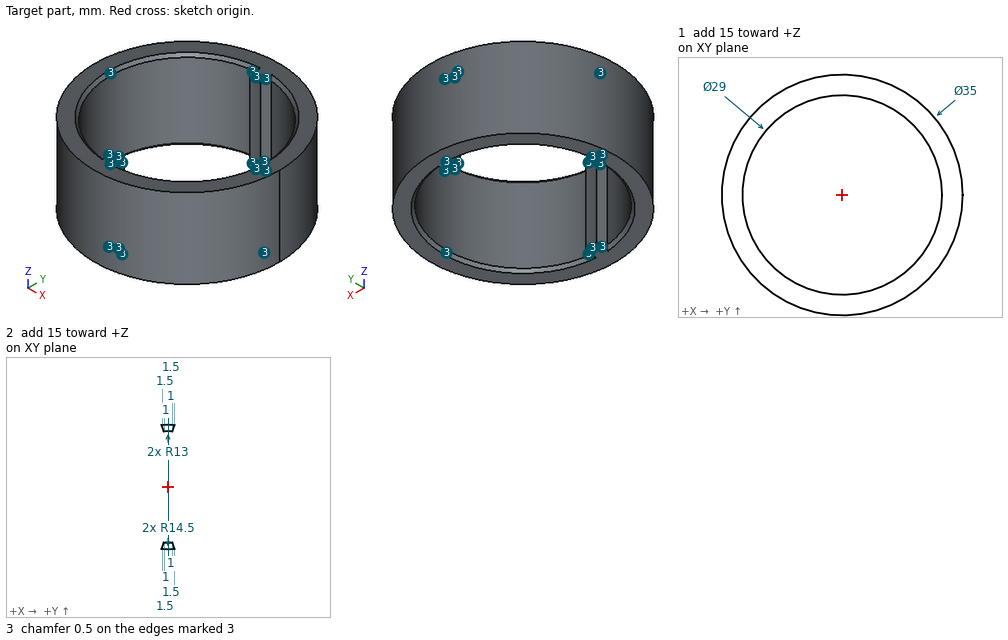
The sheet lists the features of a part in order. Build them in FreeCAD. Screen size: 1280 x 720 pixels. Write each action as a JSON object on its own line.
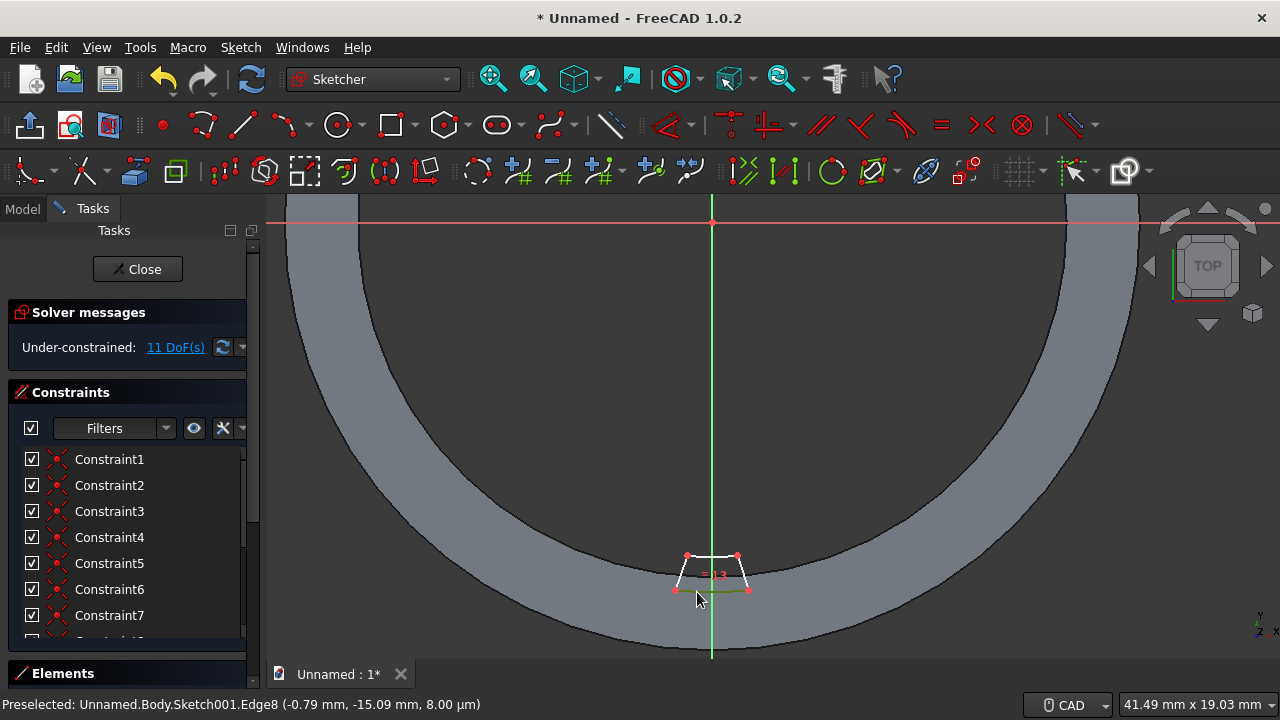
{"action": "left_click", "coordinate": [942, 126]}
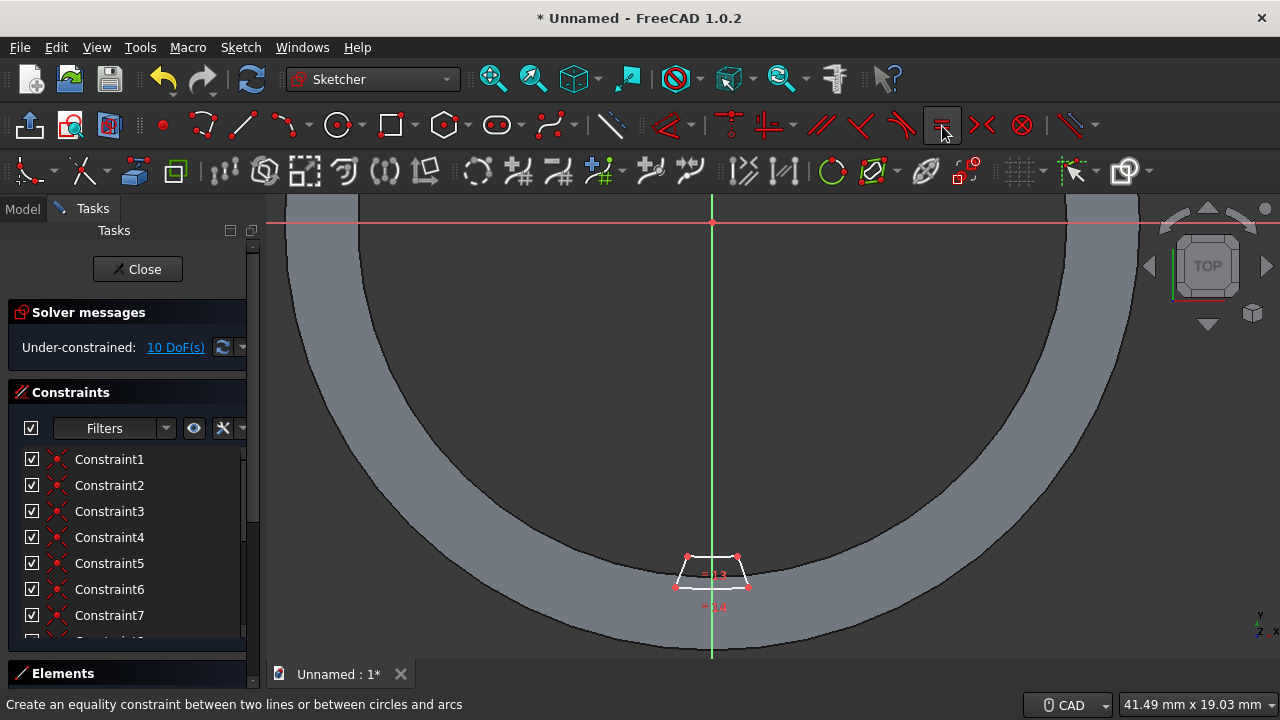
{"action": "key", "text": "d"}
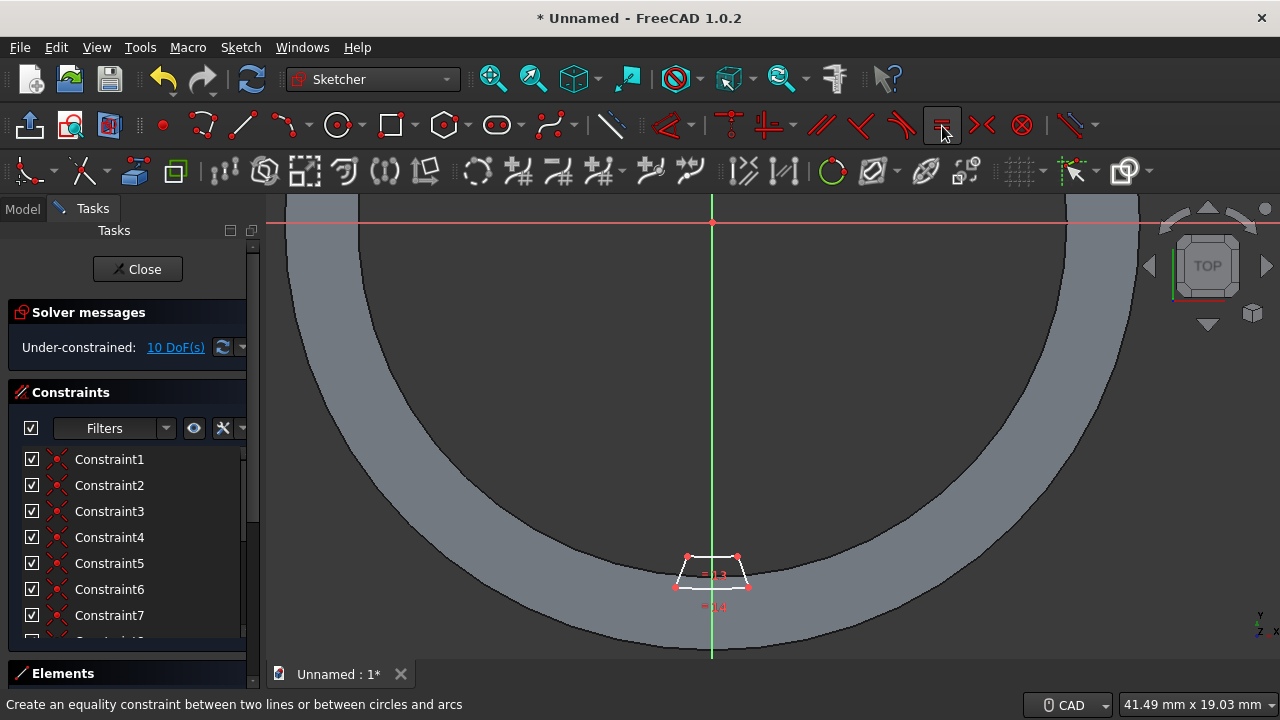
{"action": "scroll", "coordinate": [698, 593], "scroll_direction": "down", "scroll_amount": 4}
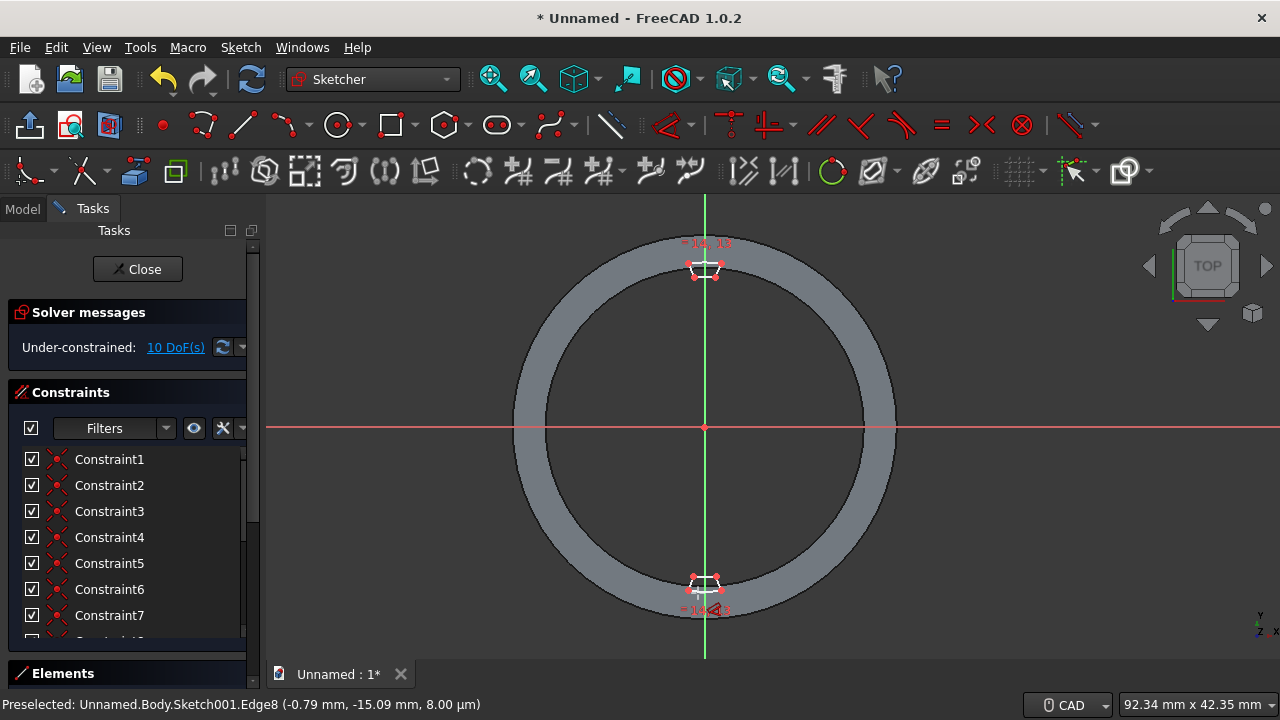
{"action": "scroll", "coordinate": [709, 277], "scroll_direction": "up", "scroll_amount": 6}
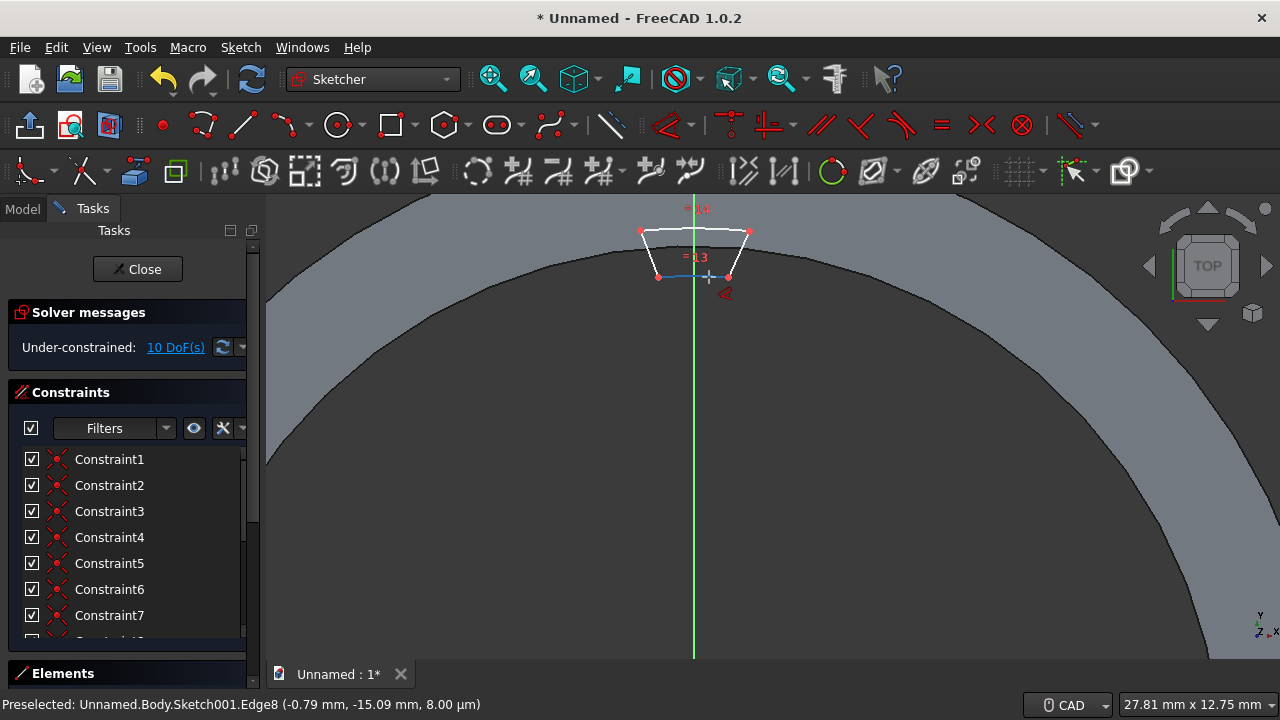
{"action": "left_click", "coordinate": [708, 276]}
{"action": "left_click", "coordinate": [709, 244]}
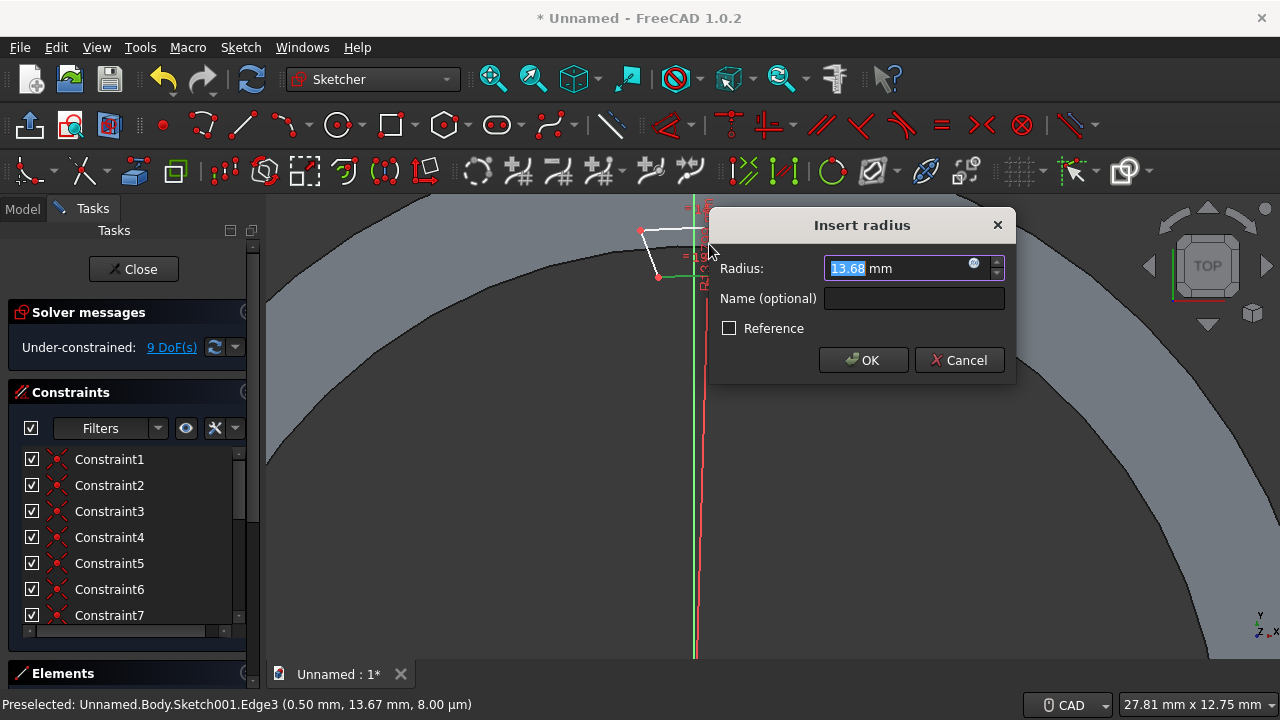
{"action": "type", "text": "13"}
{"action": "key", "text": "Return"}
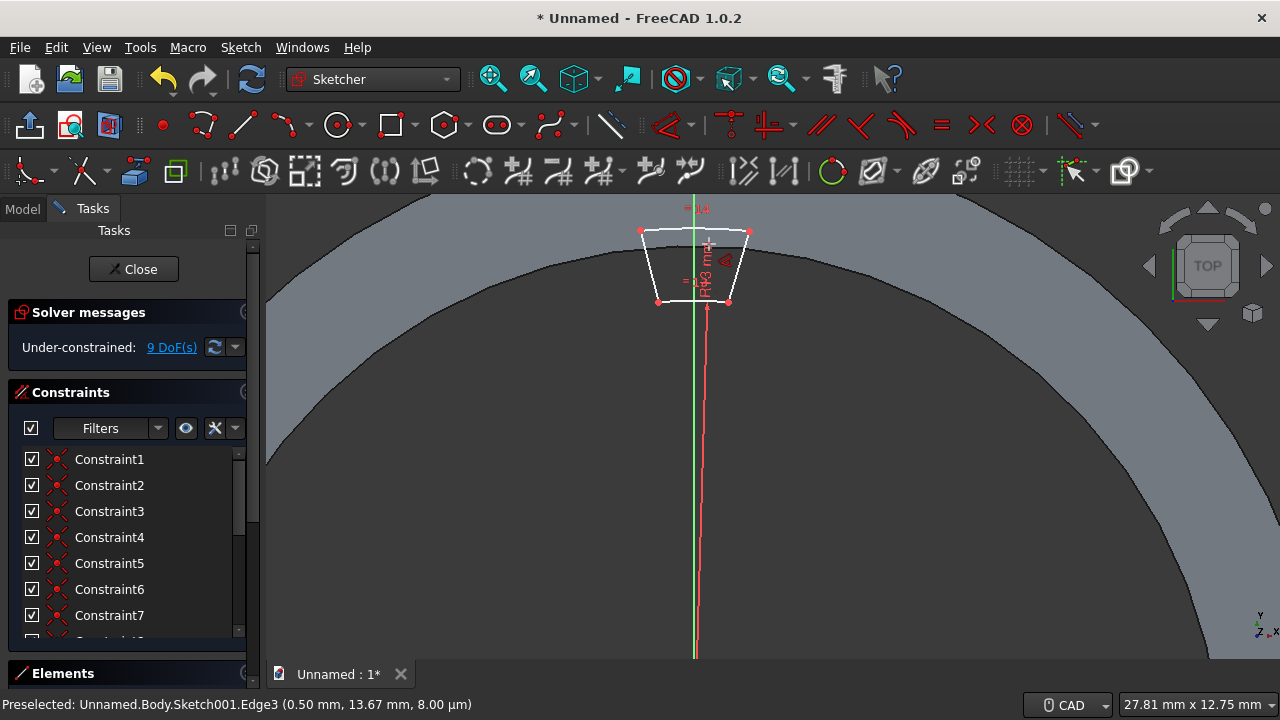
{"action": "left_click", "coordinate": [717, 229]}
{"action": "left_click", "coordinate": [992, 280]}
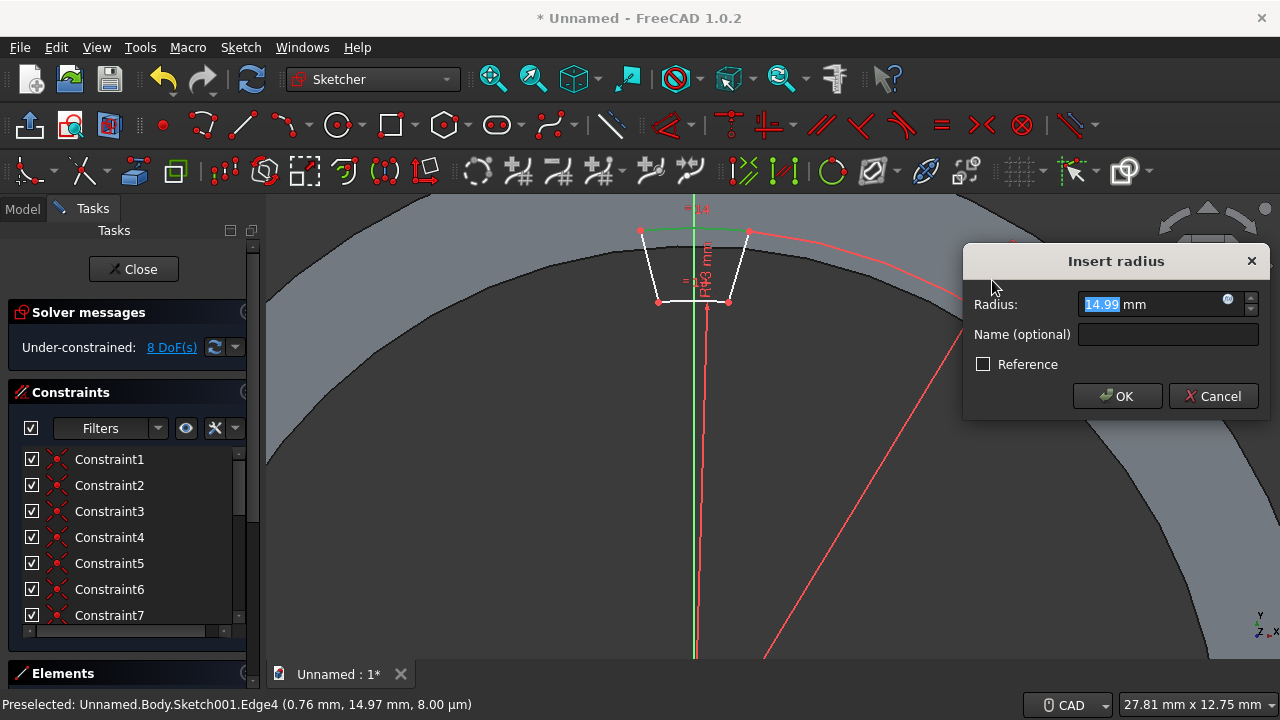
{"action": "type", "text": "14.5"}
{"action": "key", "text": "Return"}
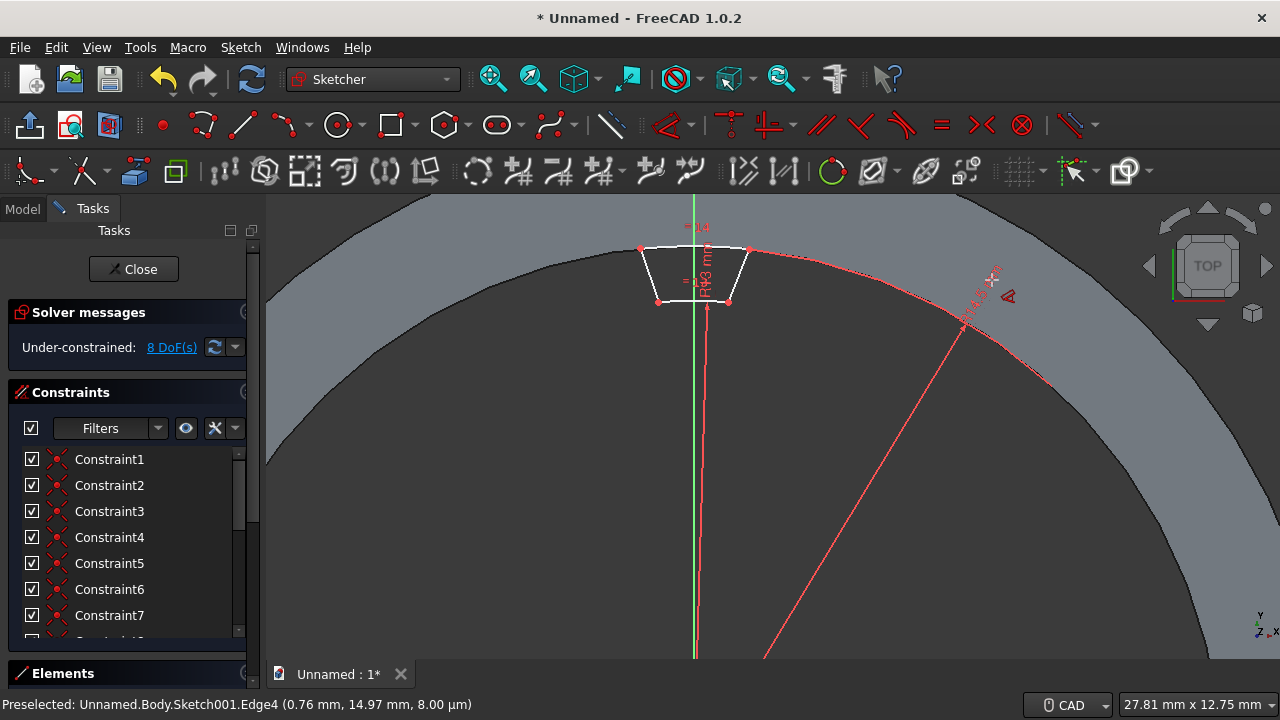
{"action": "left_click", "coordinate": [659, 302]}
{"action": "left_click", "coordinate": [676, 268]}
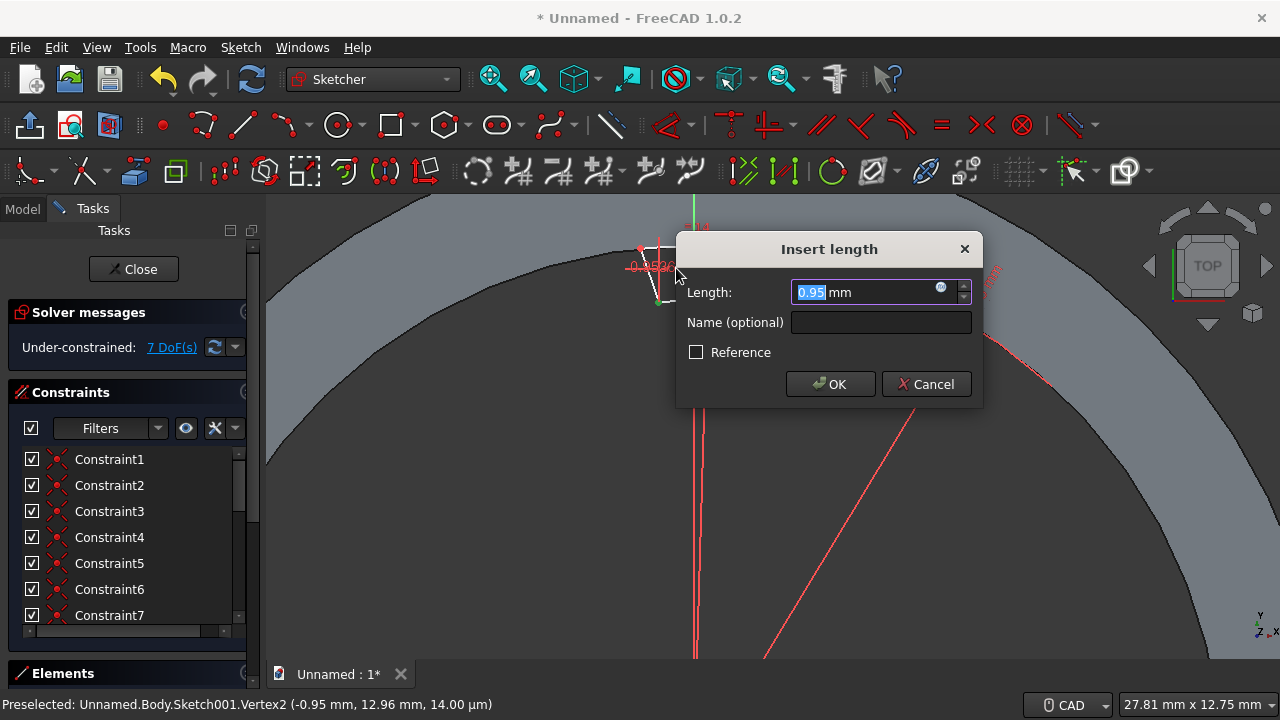
{"action": "type", "text": "1"}
{"action": "key", "text": "Return"}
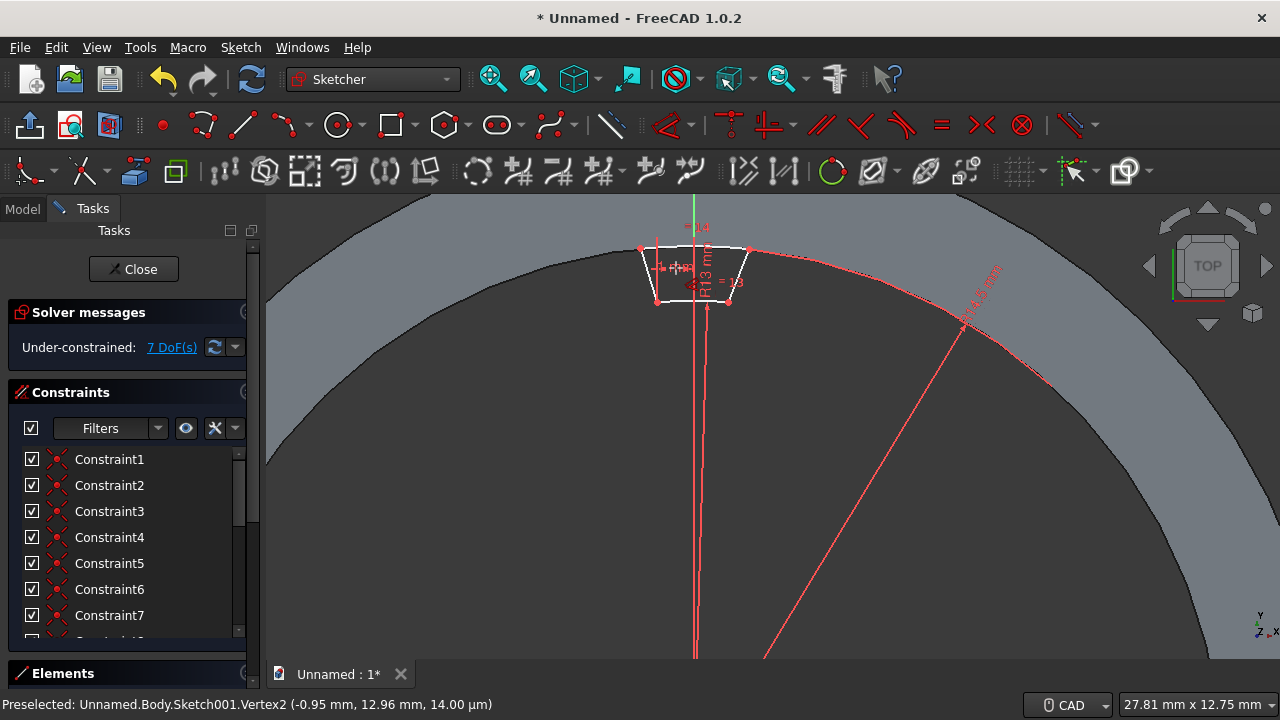
{"action": "left_click", "coordinate": [728, 302]}
{"action": "left_click", "coordinate": [719, 268]}